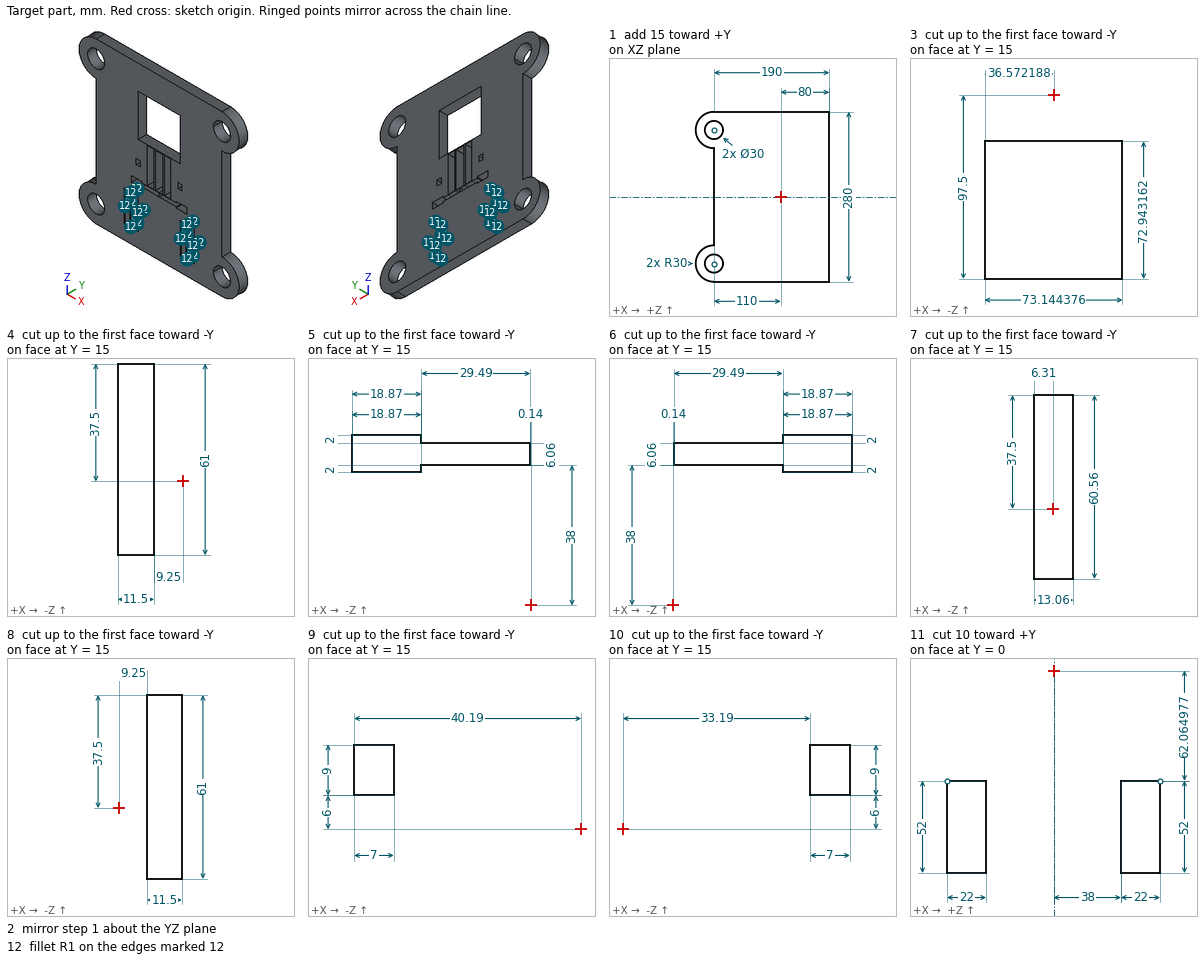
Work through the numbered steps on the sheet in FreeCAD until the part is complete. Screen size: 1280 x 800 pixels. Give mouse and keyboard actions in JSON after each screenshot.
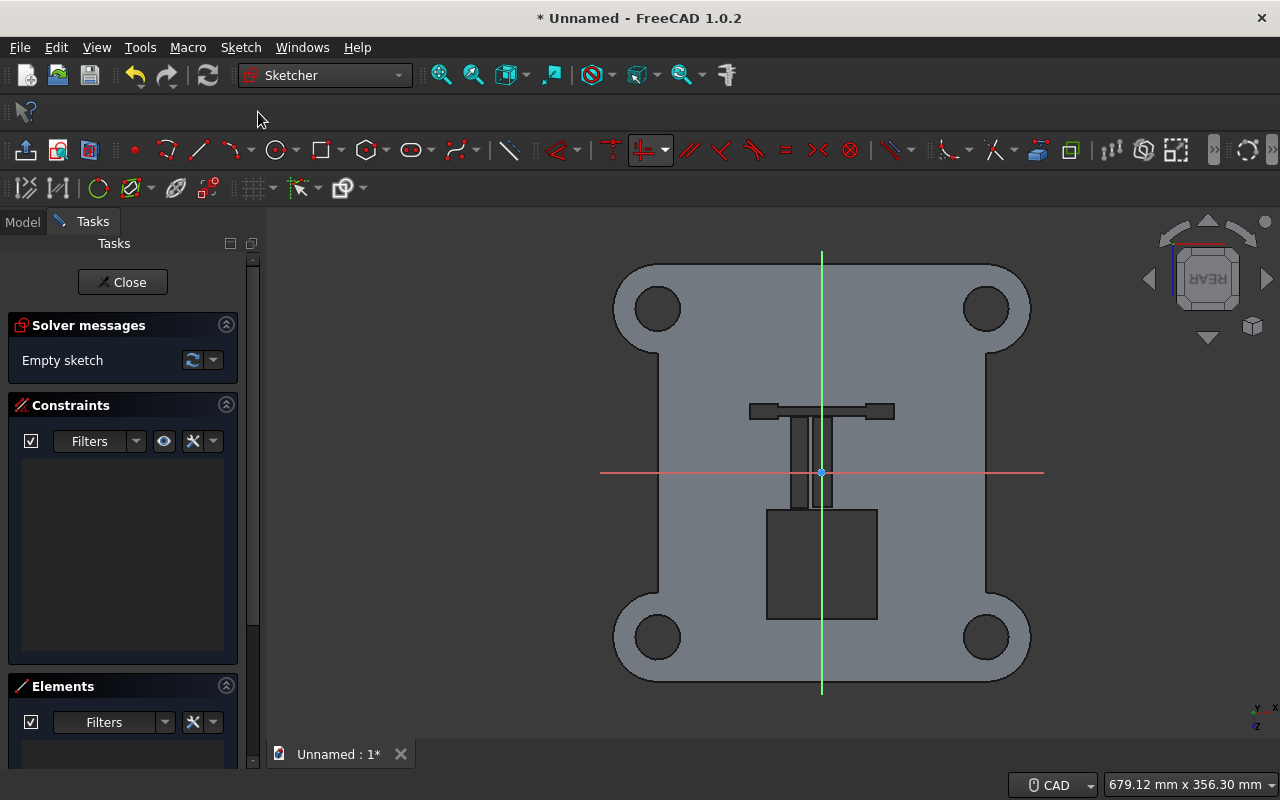
{"action": "scroll", "coordinate": [881, 459], "scroll_direction": "up", "scroll_amount": 7}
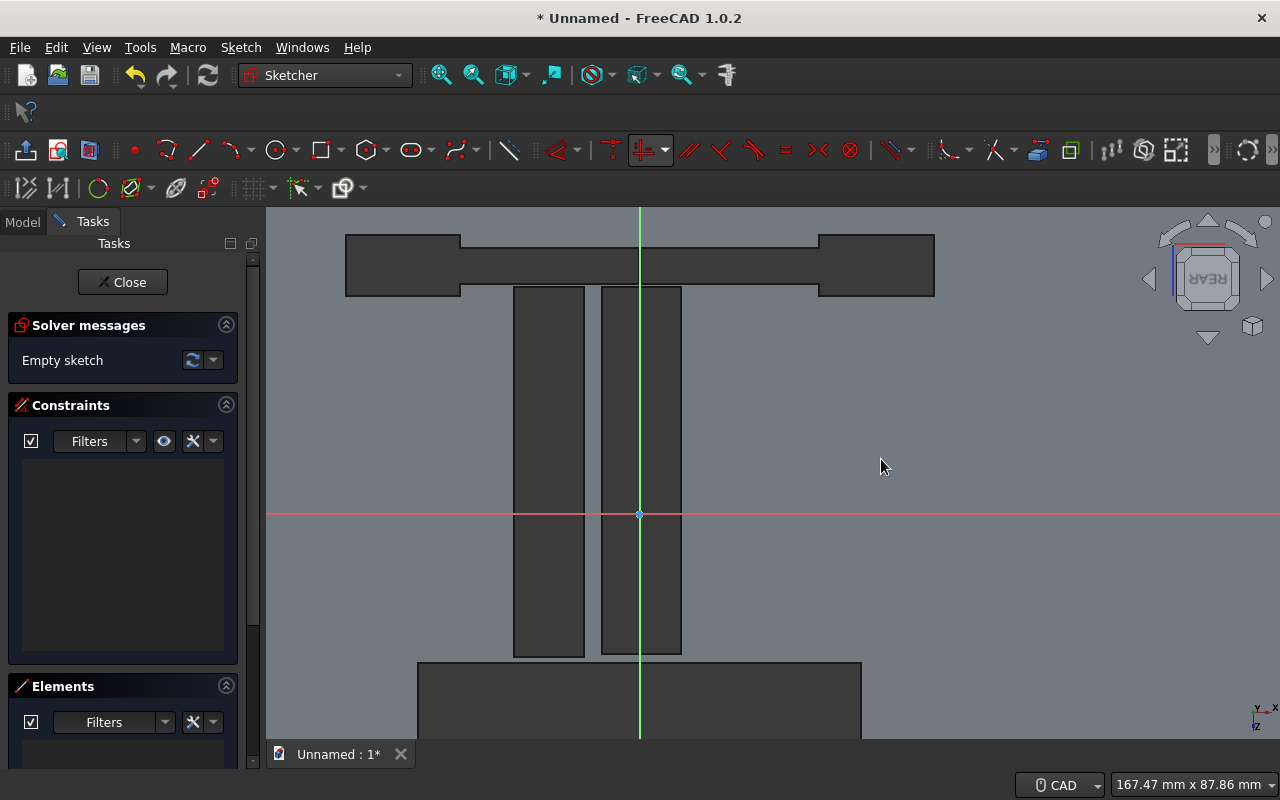
{"action": "left_click", "coordinate": [322, 150]}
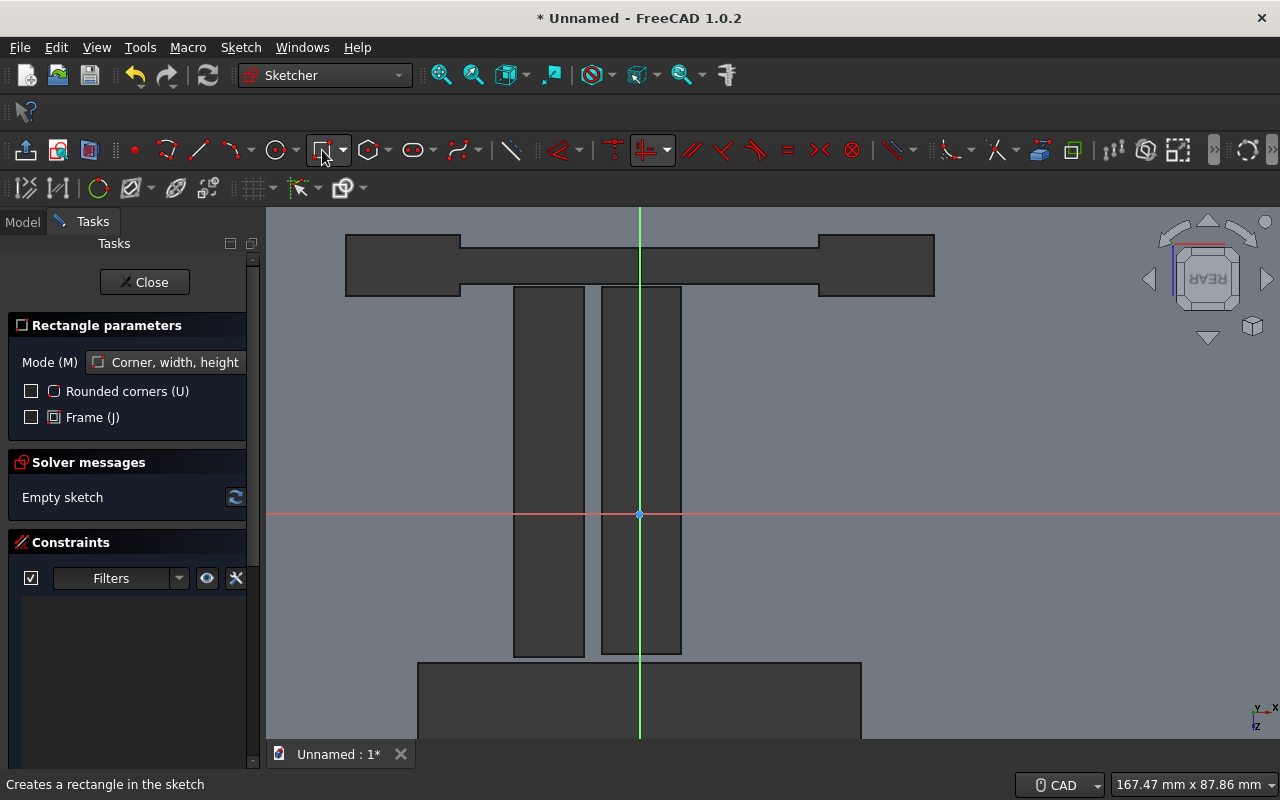
{"action": "left_click", "coordinate": [696, 287]}
{"action": "mouse_move", "coordinate": [766, 657]}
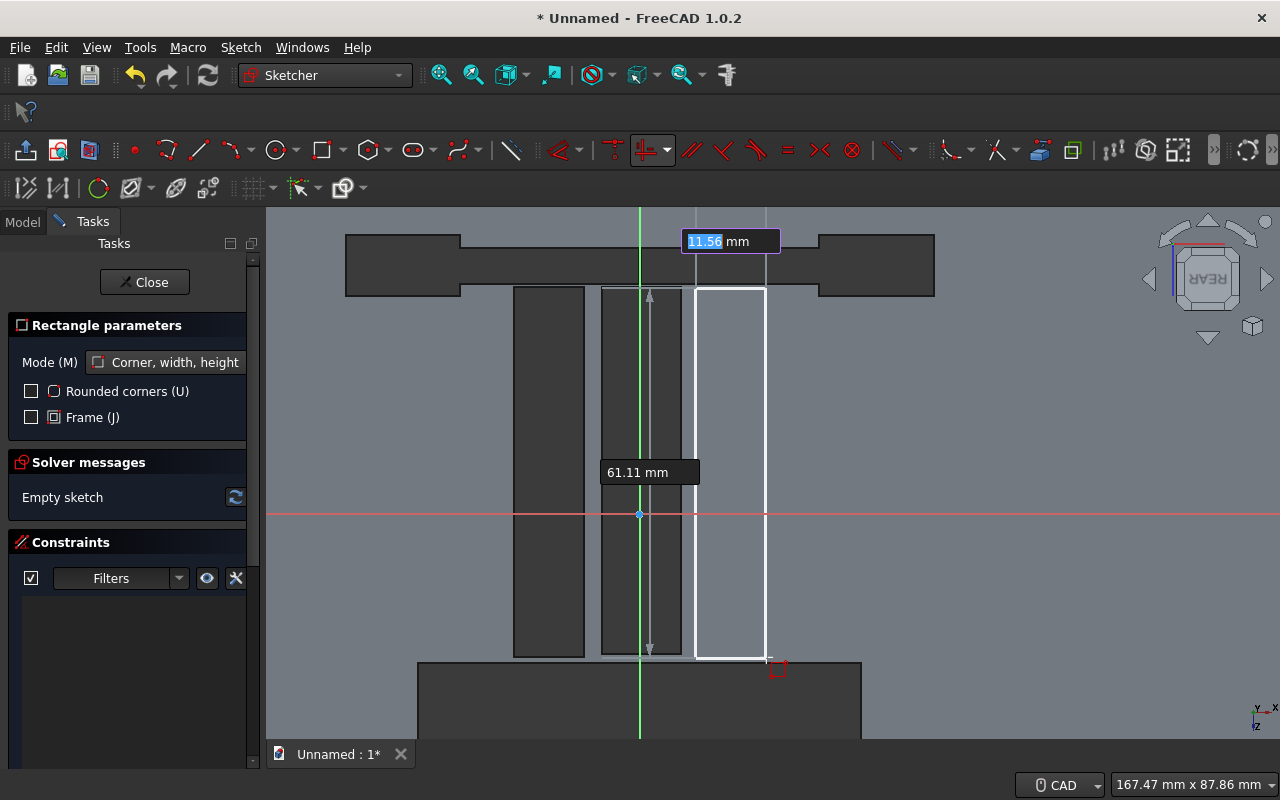
{"action": "type", "text": "11.5"}
{"action": "key", "text": "Tab"}
{"action": "type", "text": "61"}
{"action": "key", "text": "Return"}
{"action": "key", "text": "Escape"}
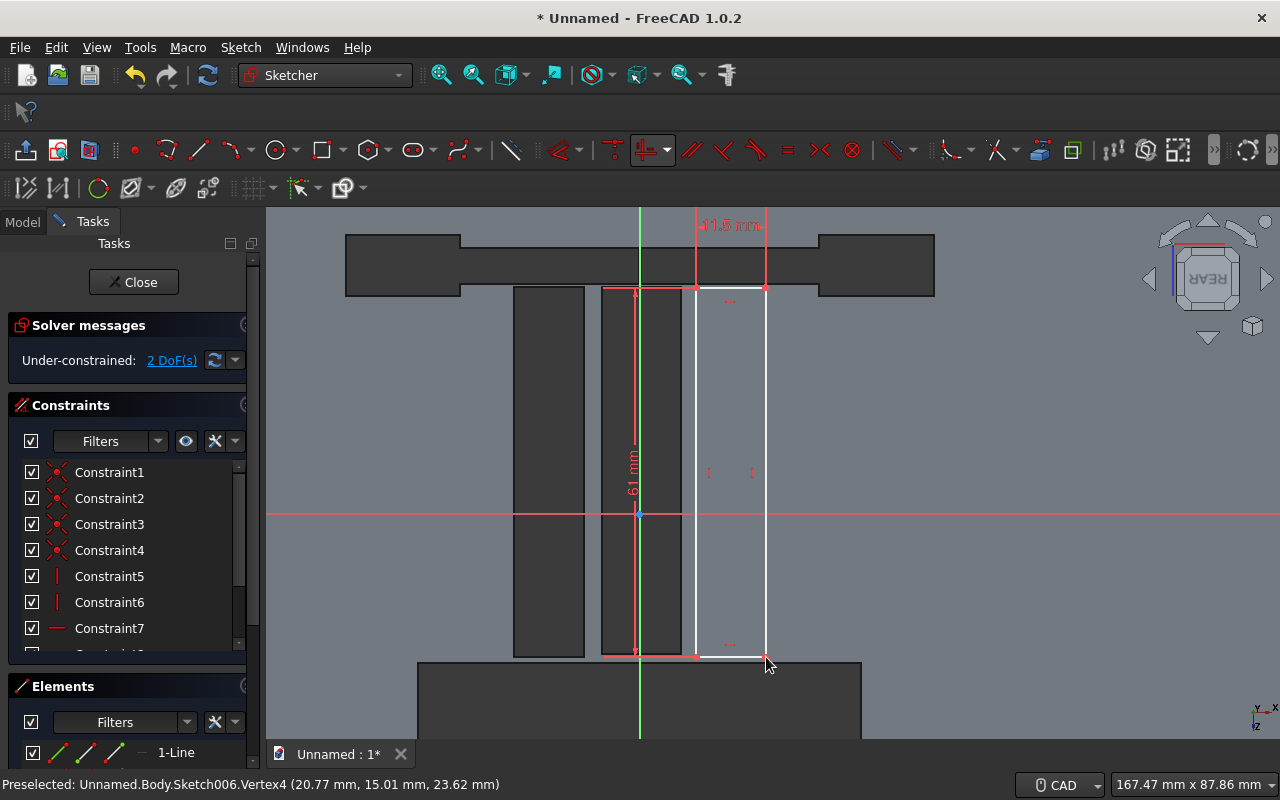
{"action": "key", "text": "d"}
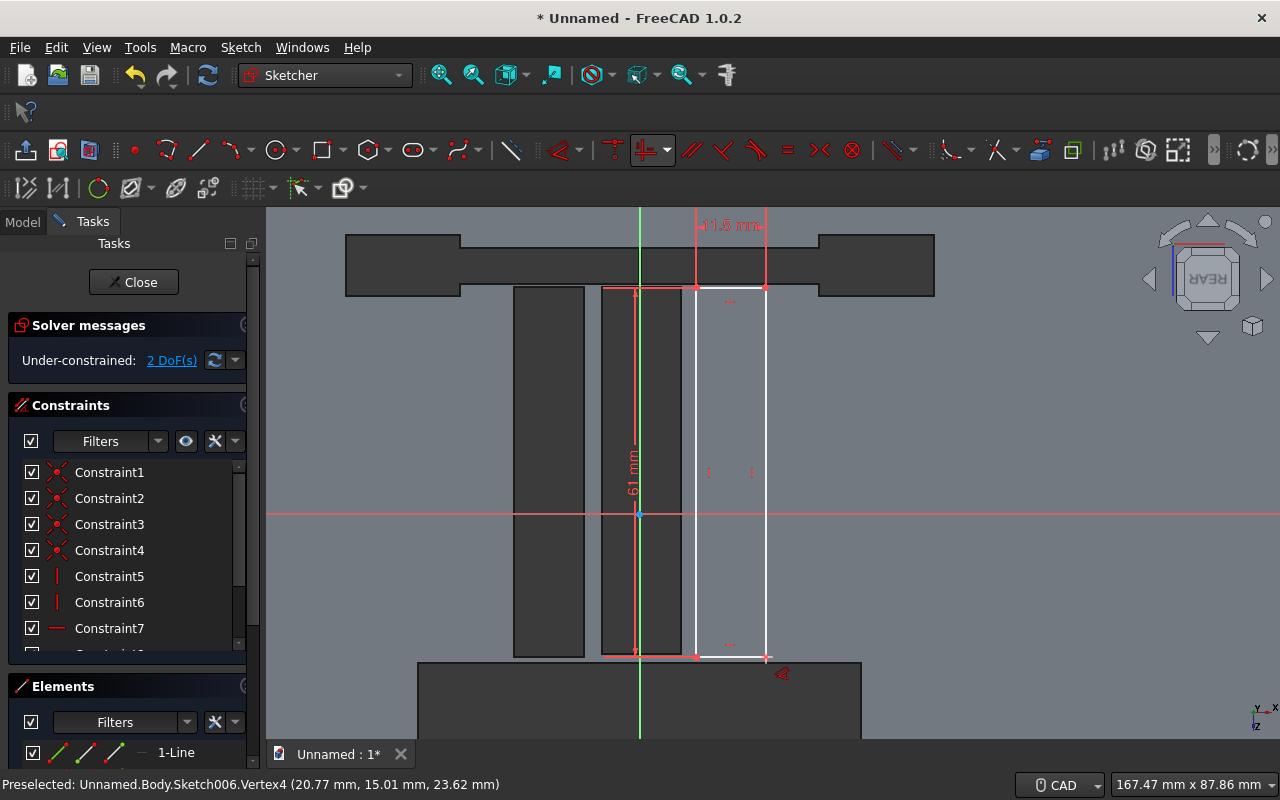
{"action": "left_click", "coordinate": [696, 288]}
{"action": "left_click", "coordinate": [668, 254]}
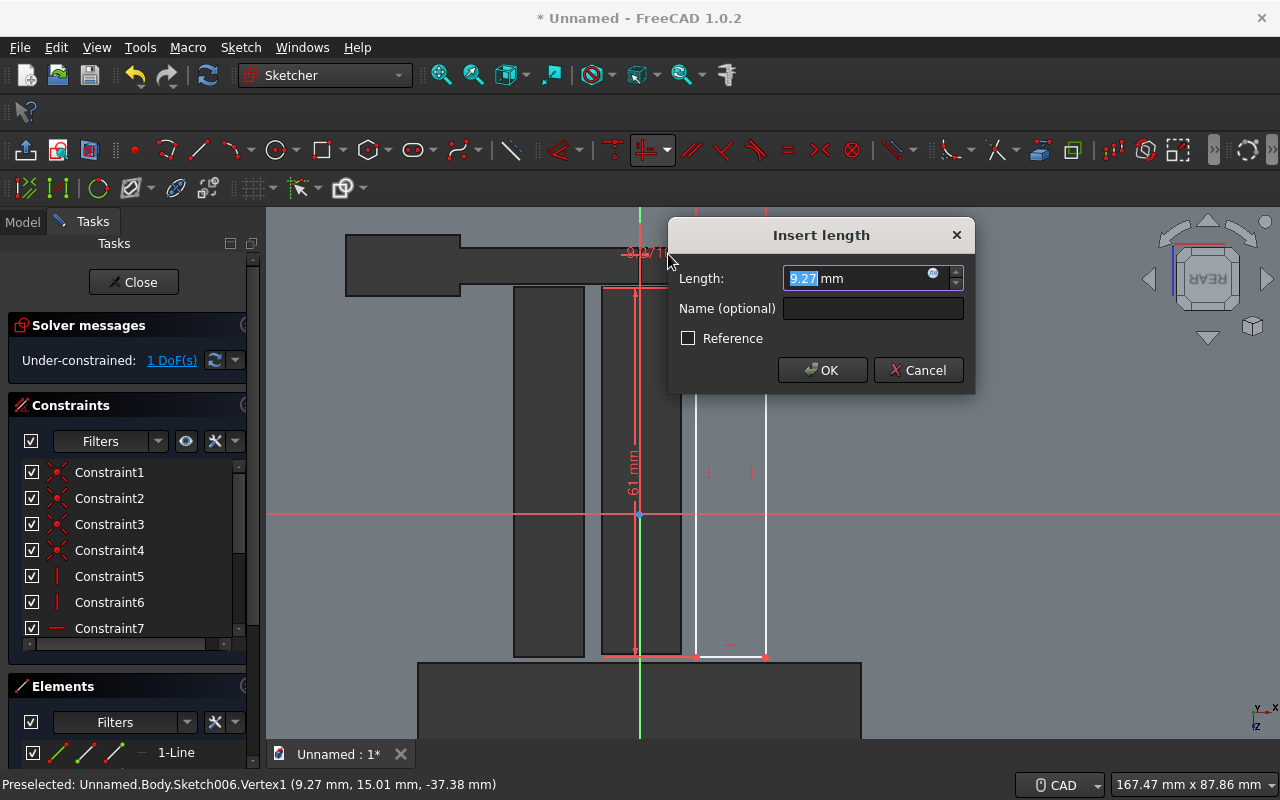
{"action": "type", "text": "9.25"}
{"action": "key", "text": "Return"}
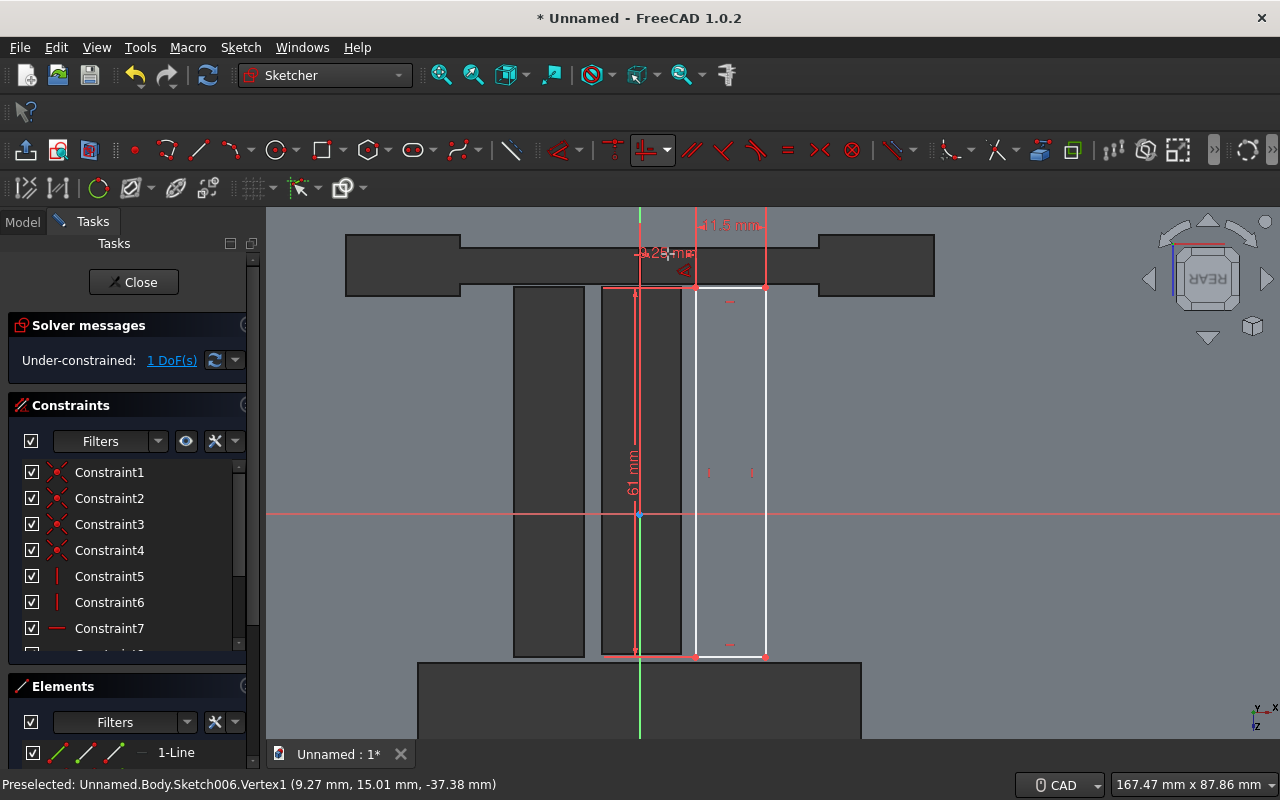
{"action": "left_click", "coordinate": [696, 288]}
{"action": "left_click", "coordinate": [606, 401]}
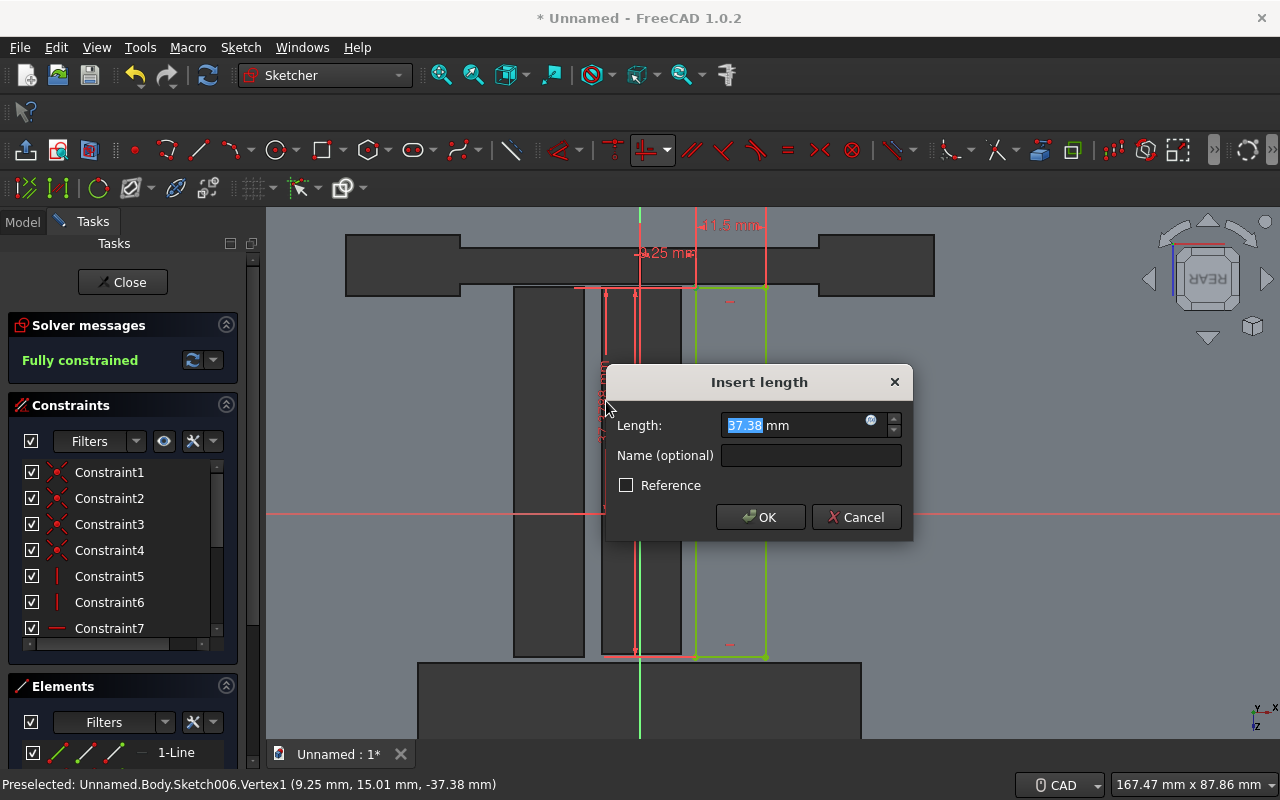
{"action": "type", "text": "37.5"}
{"action": "key", "text": "Return"}
{"action": "key", "text": "Escape"}